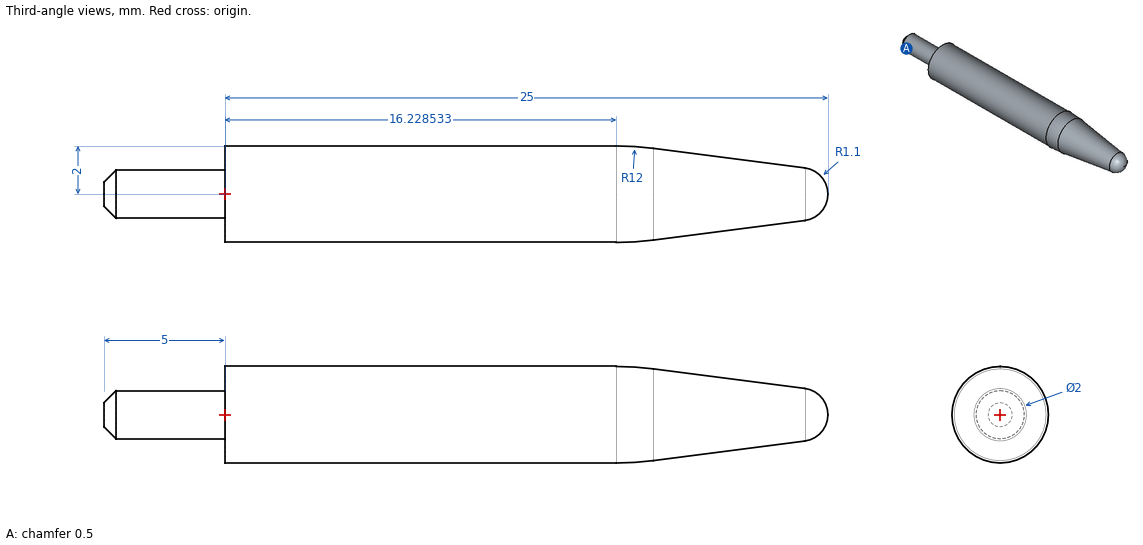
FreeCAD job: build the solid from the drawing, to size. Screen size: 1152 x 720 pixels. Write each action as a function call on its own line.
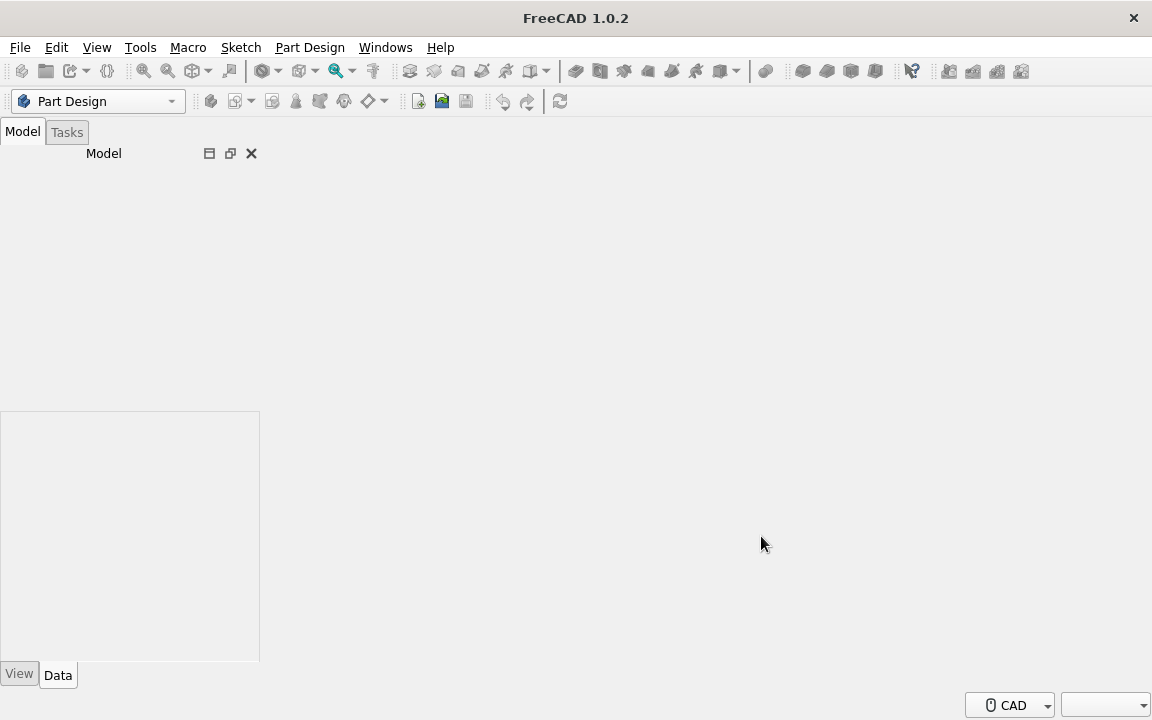
key(ctrl+n)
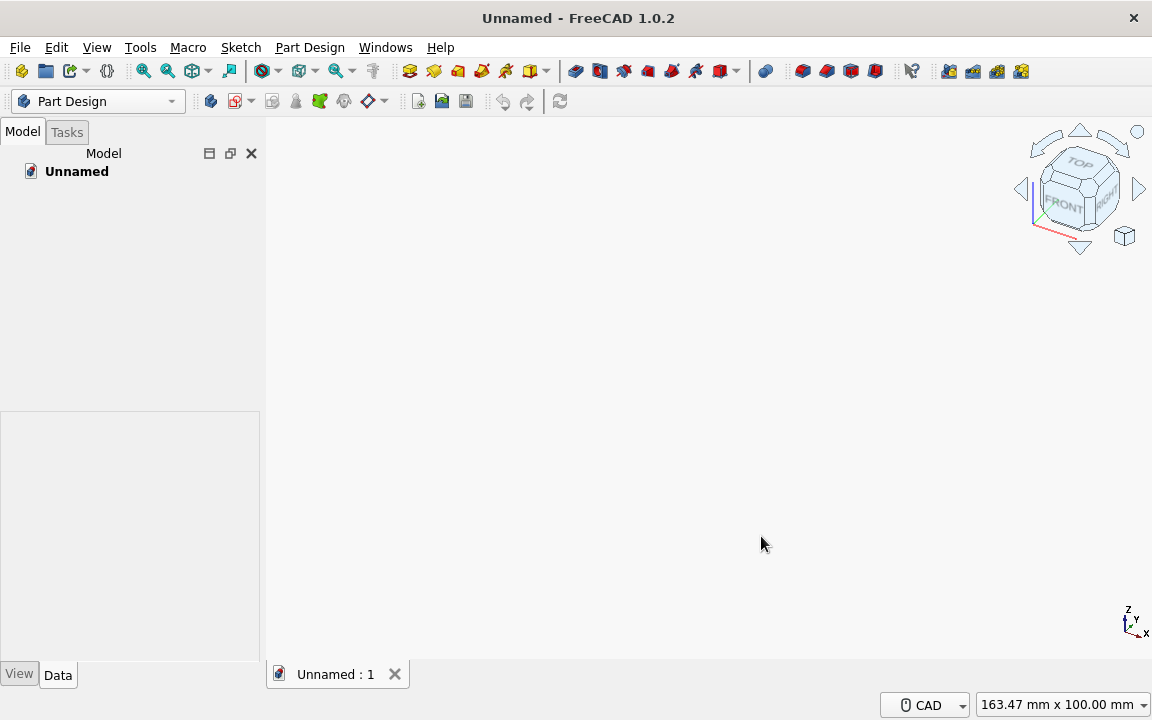
click(236, 102)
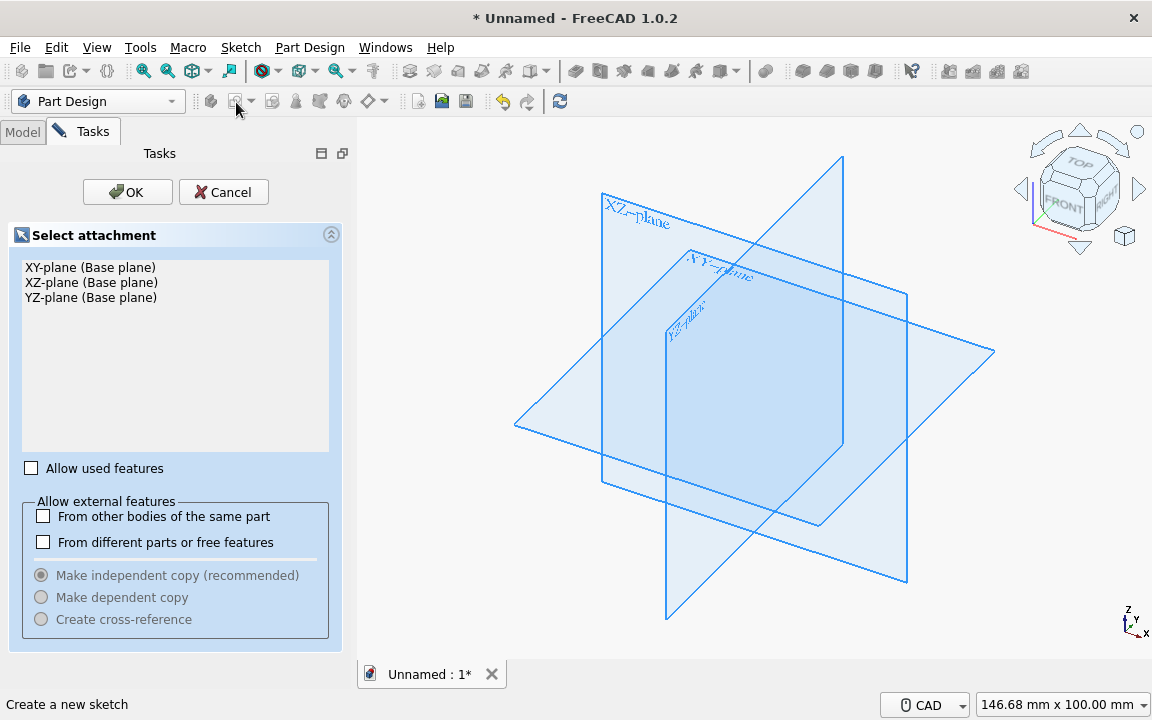
click(82, 268)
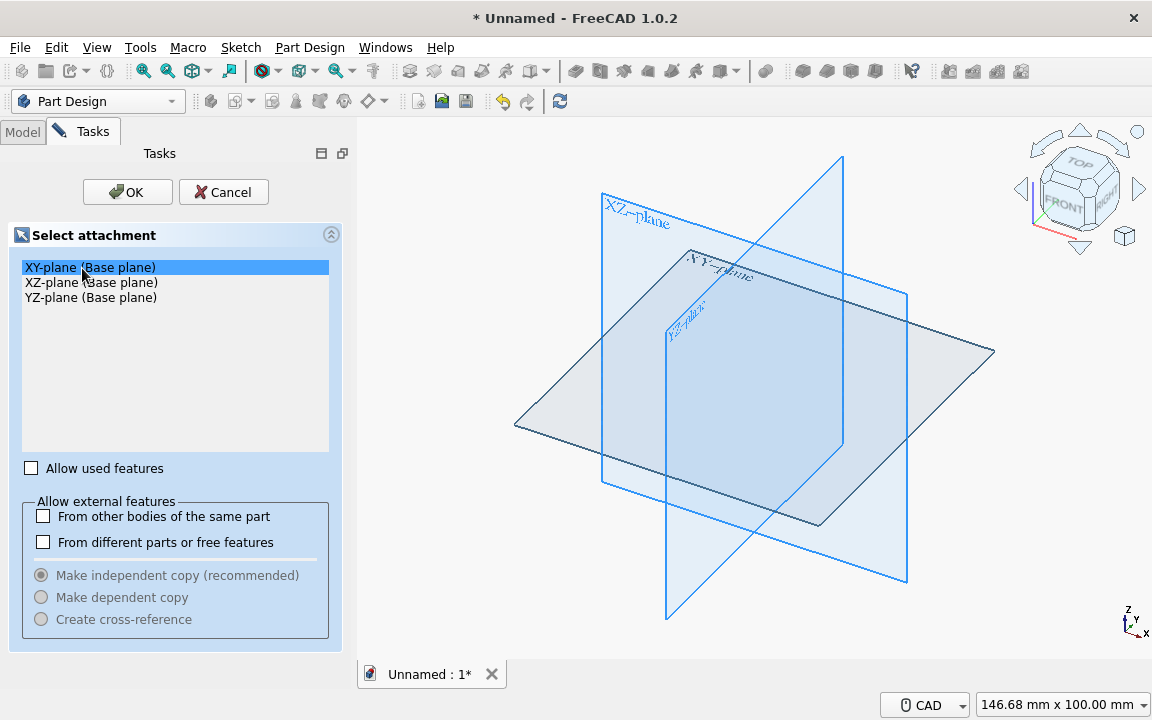
click(128, 192)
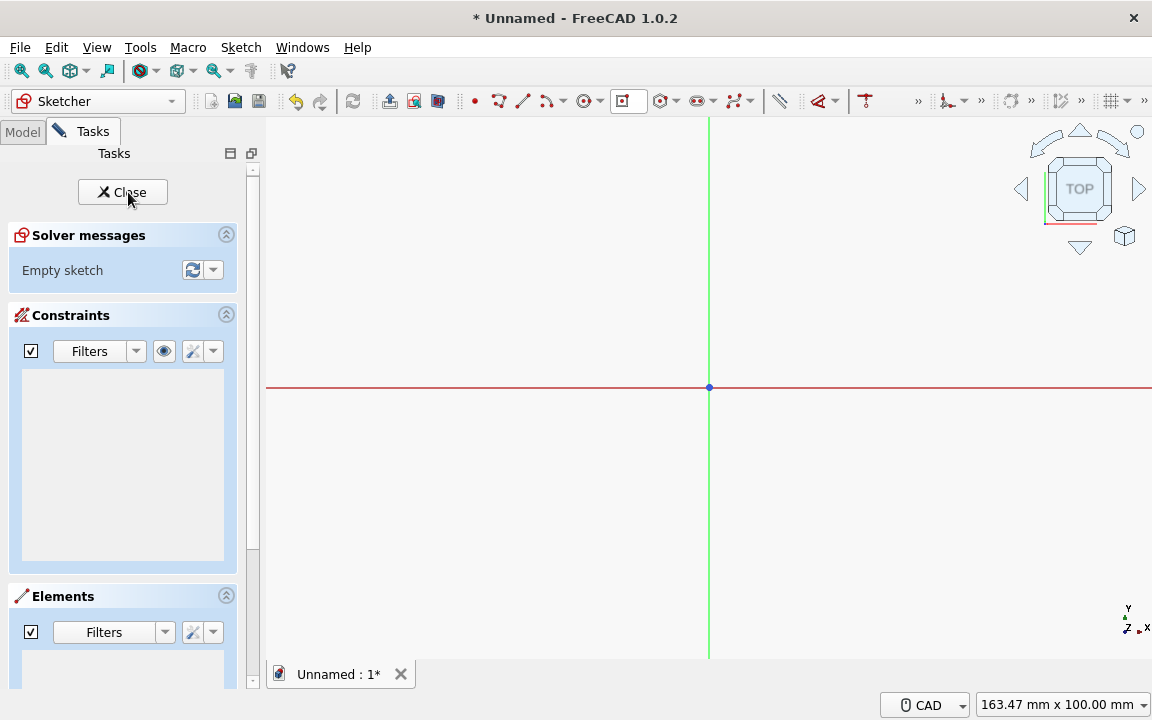
scroll(835, 380, up, 6)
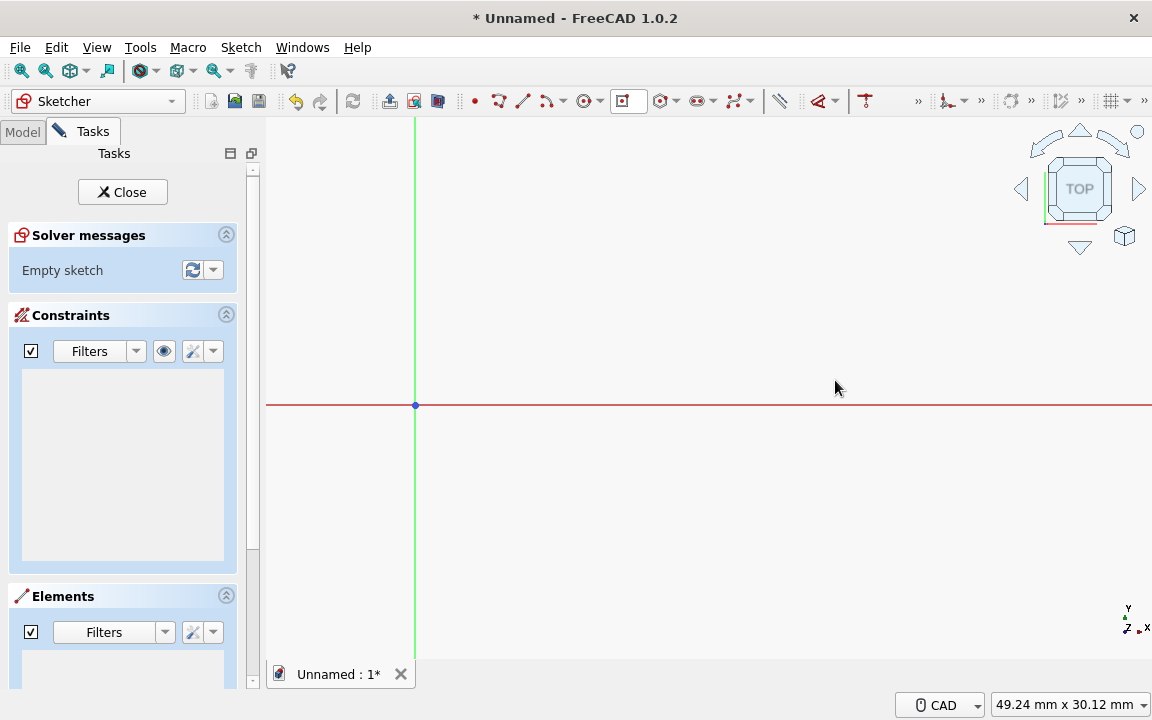
key(g)
key(l)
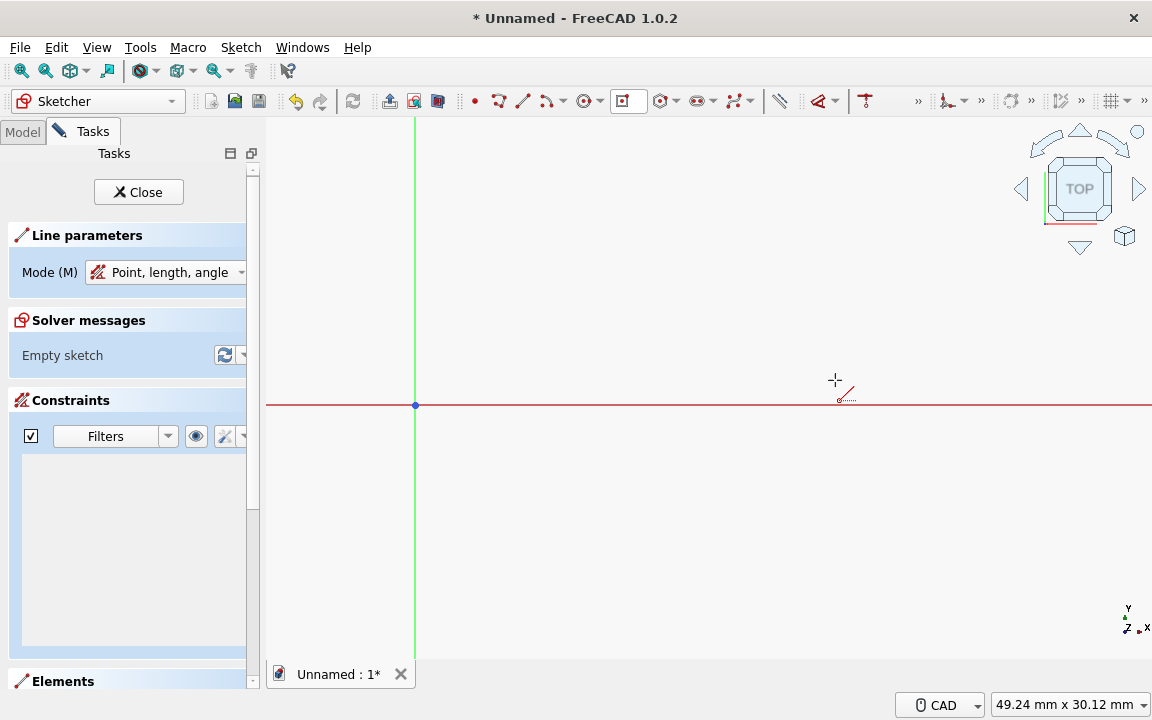
click(848, 386)
click(735, 371)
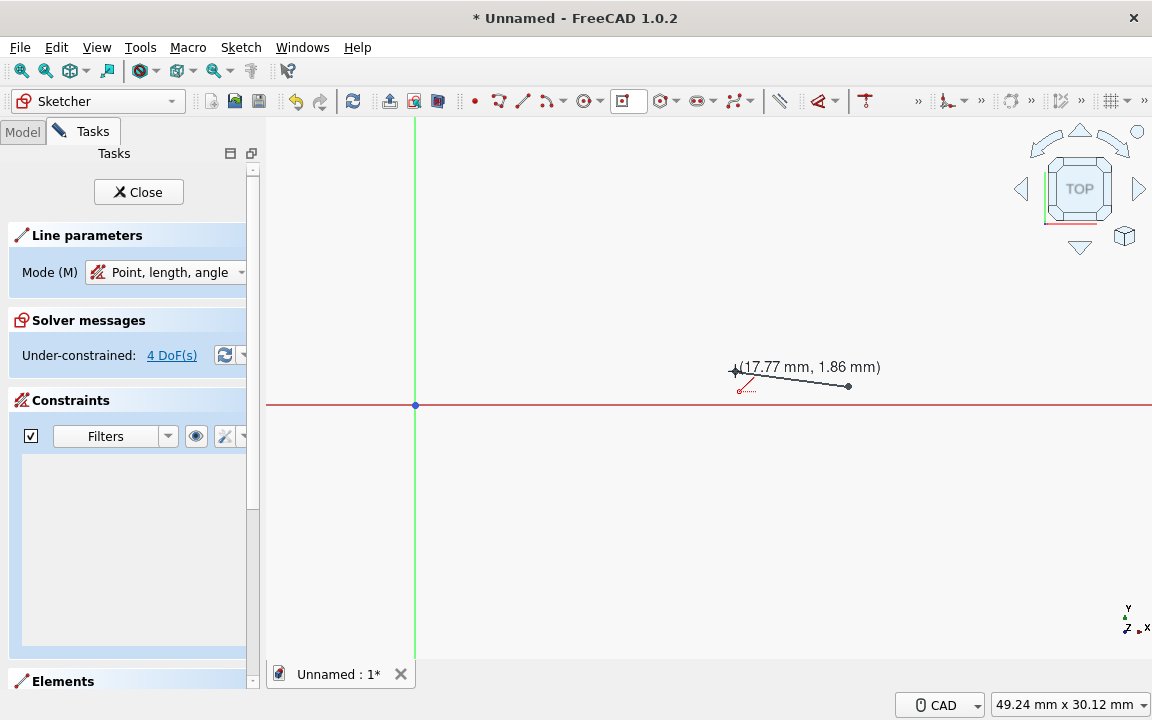
click(500, 102)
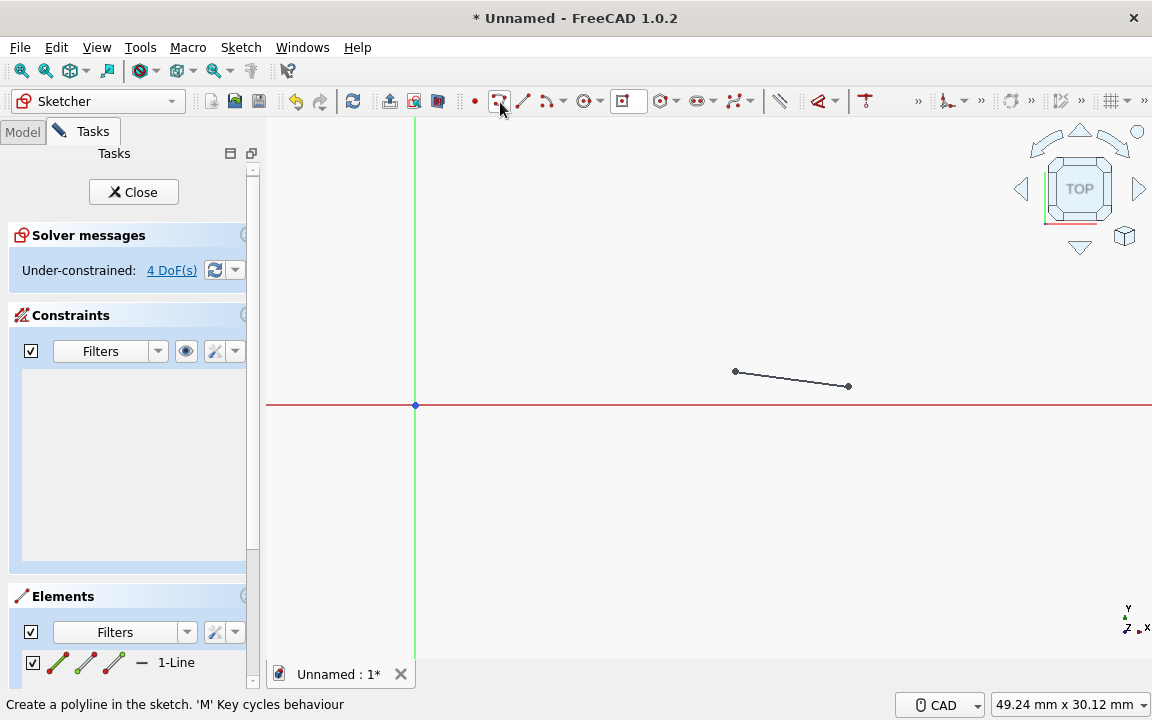
click(707, 369)
click(415, 369)
click(415, 405)
click(865, 396)
right_click(865, 396)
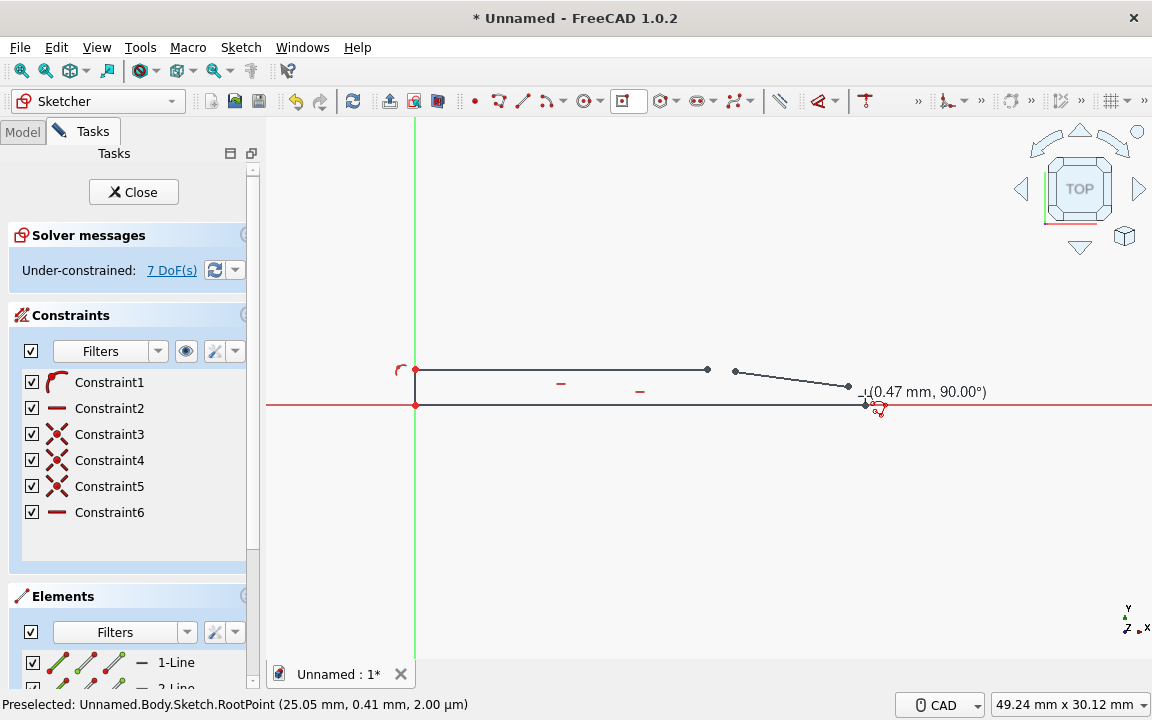
key(g)
key(3)
key(a)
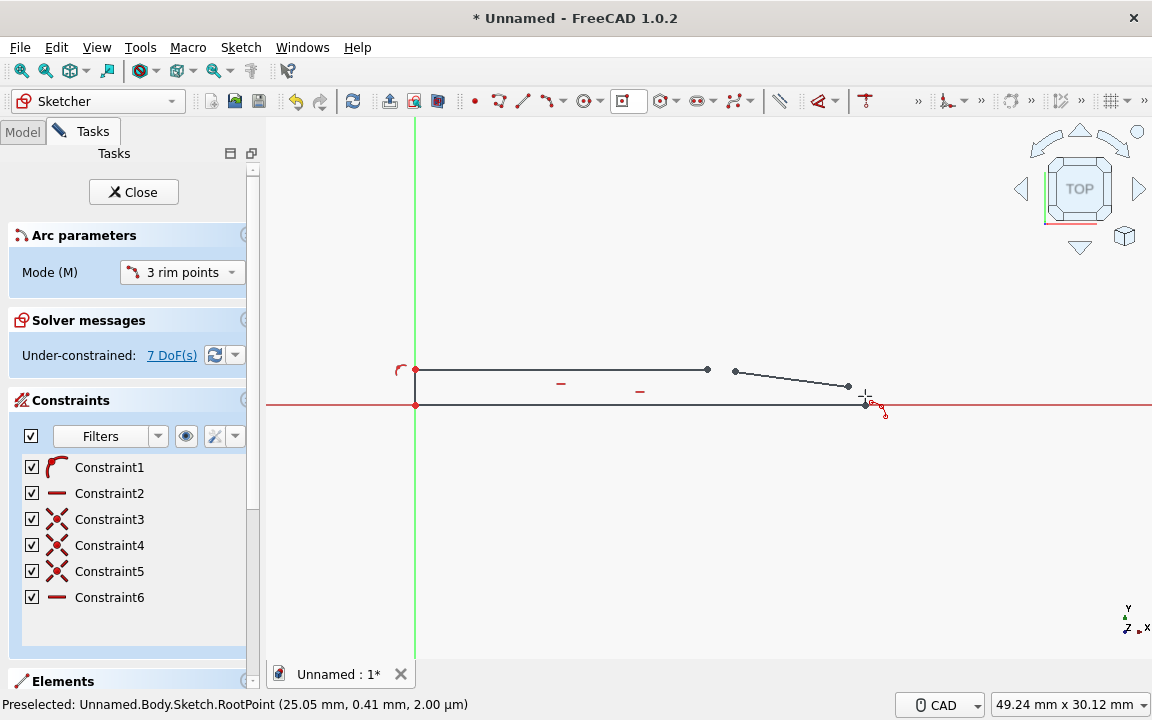
click(735, 372)
click(707, 370)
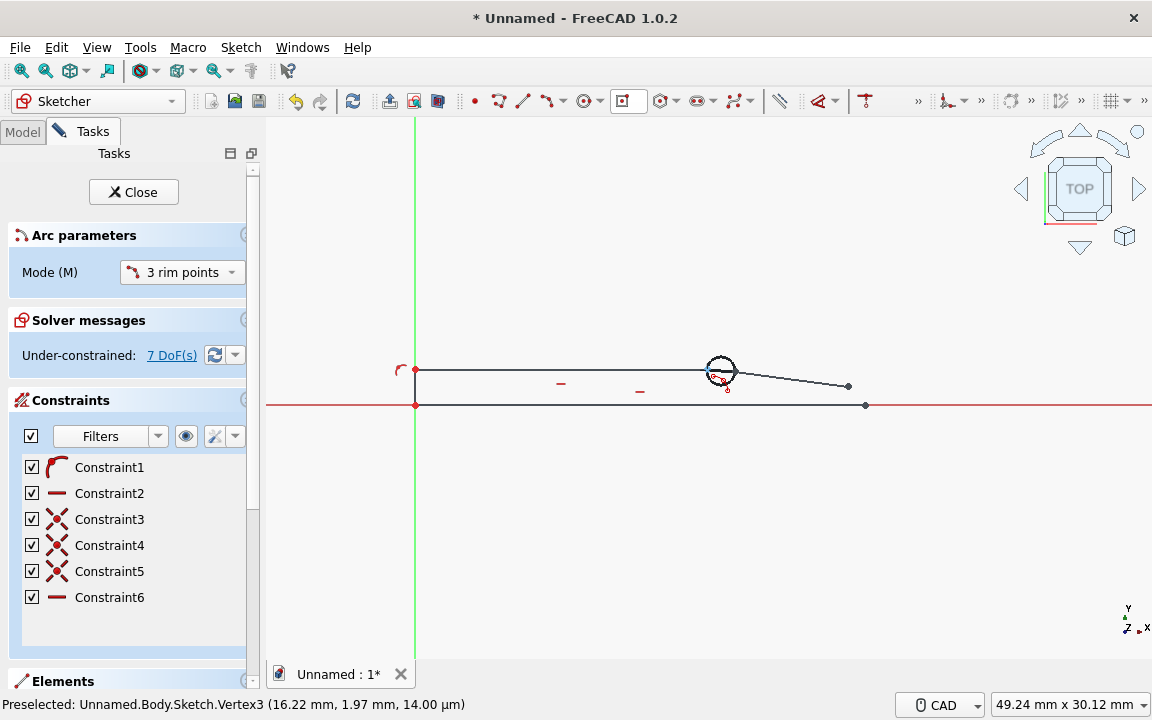
scroll(721, 370, up, 18)